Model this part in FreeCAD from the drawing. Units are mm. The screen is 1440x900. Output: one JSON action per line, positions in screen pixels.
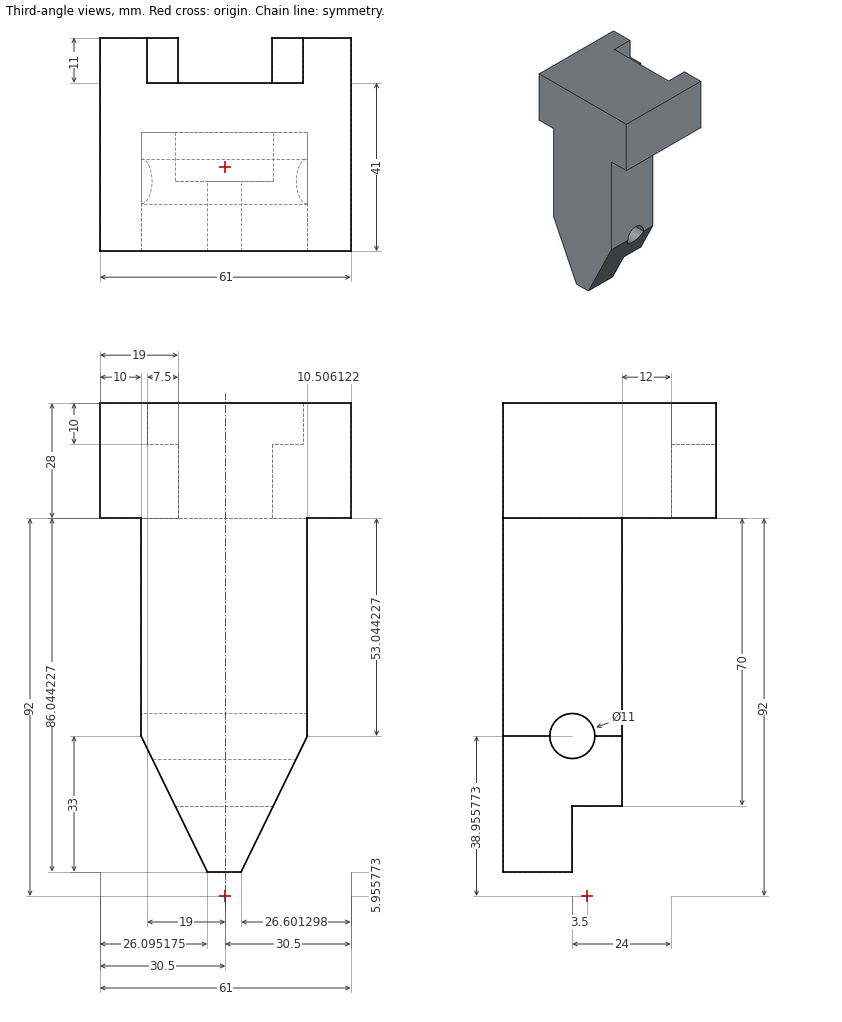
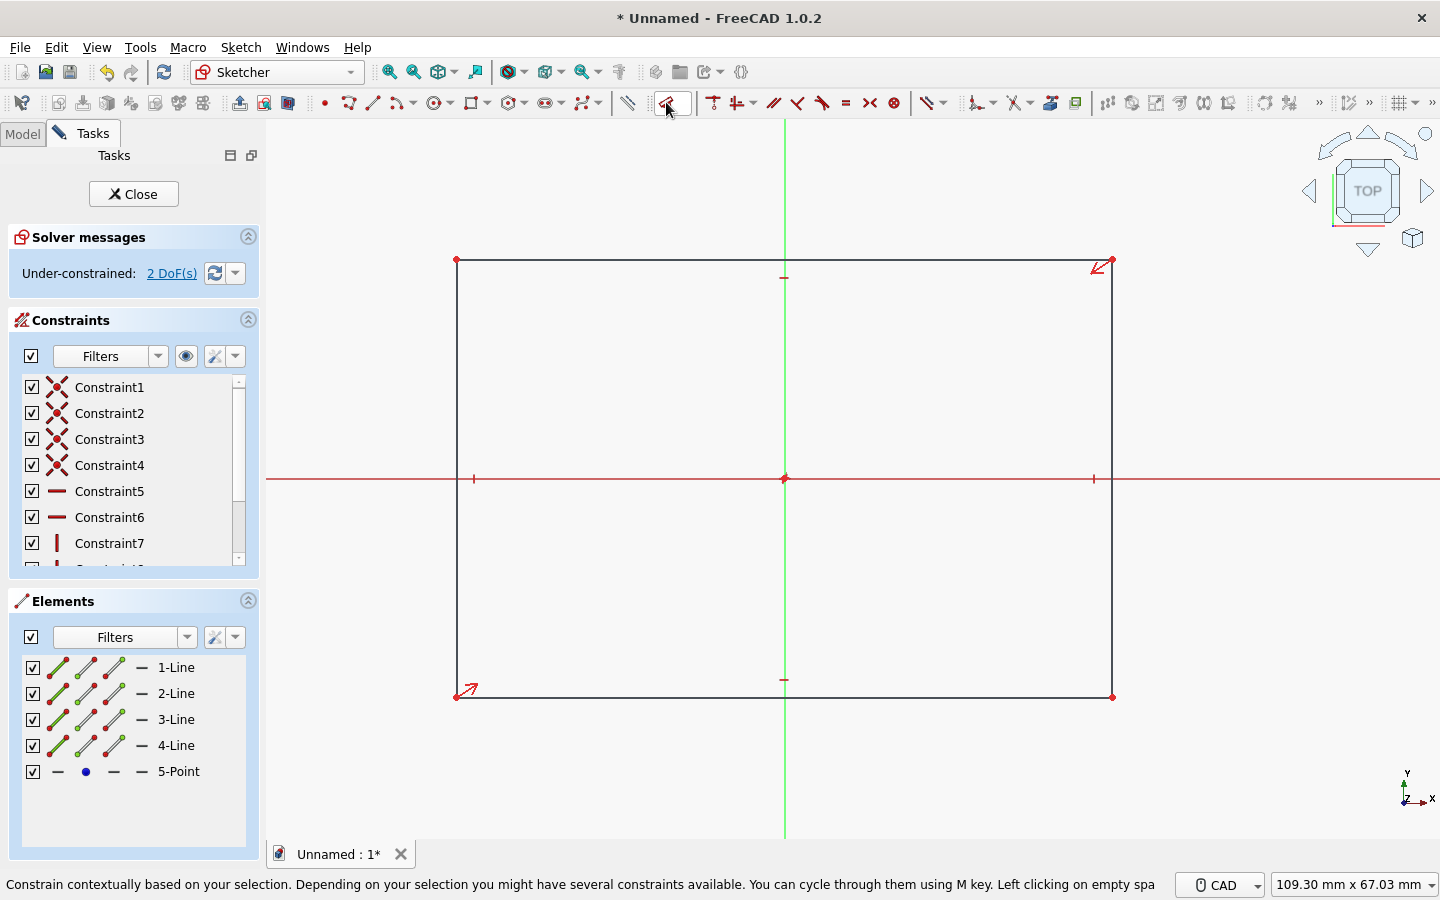
{"action": "left_click", "coordinate": [653, 698]}
{"action": "left_click", "coordinate": [634, 732]}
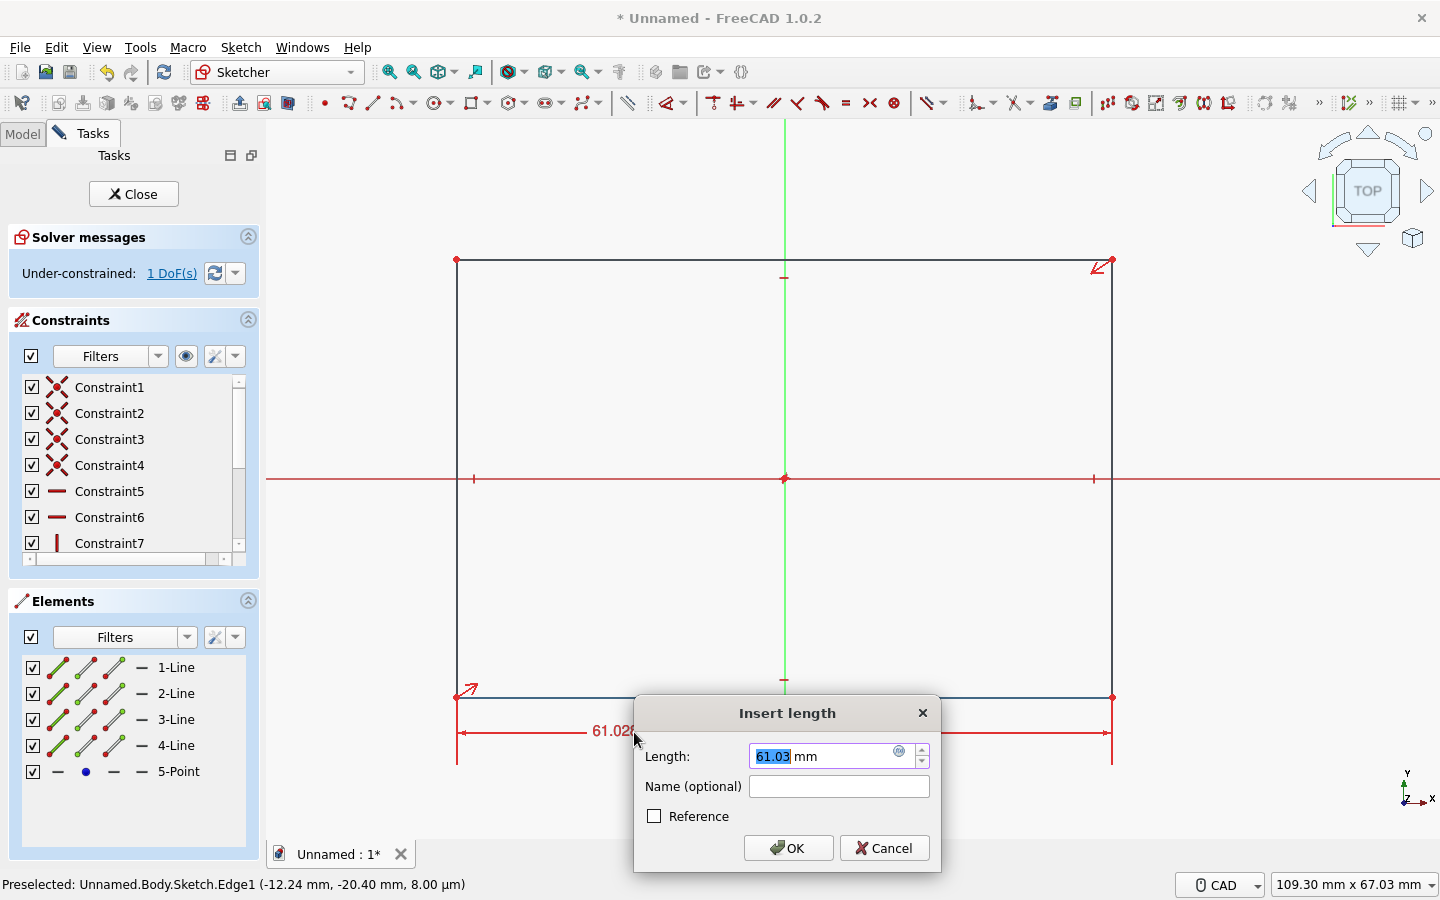
{"action": "type", "text": "61"}
{"action": "key", "text": "Return"}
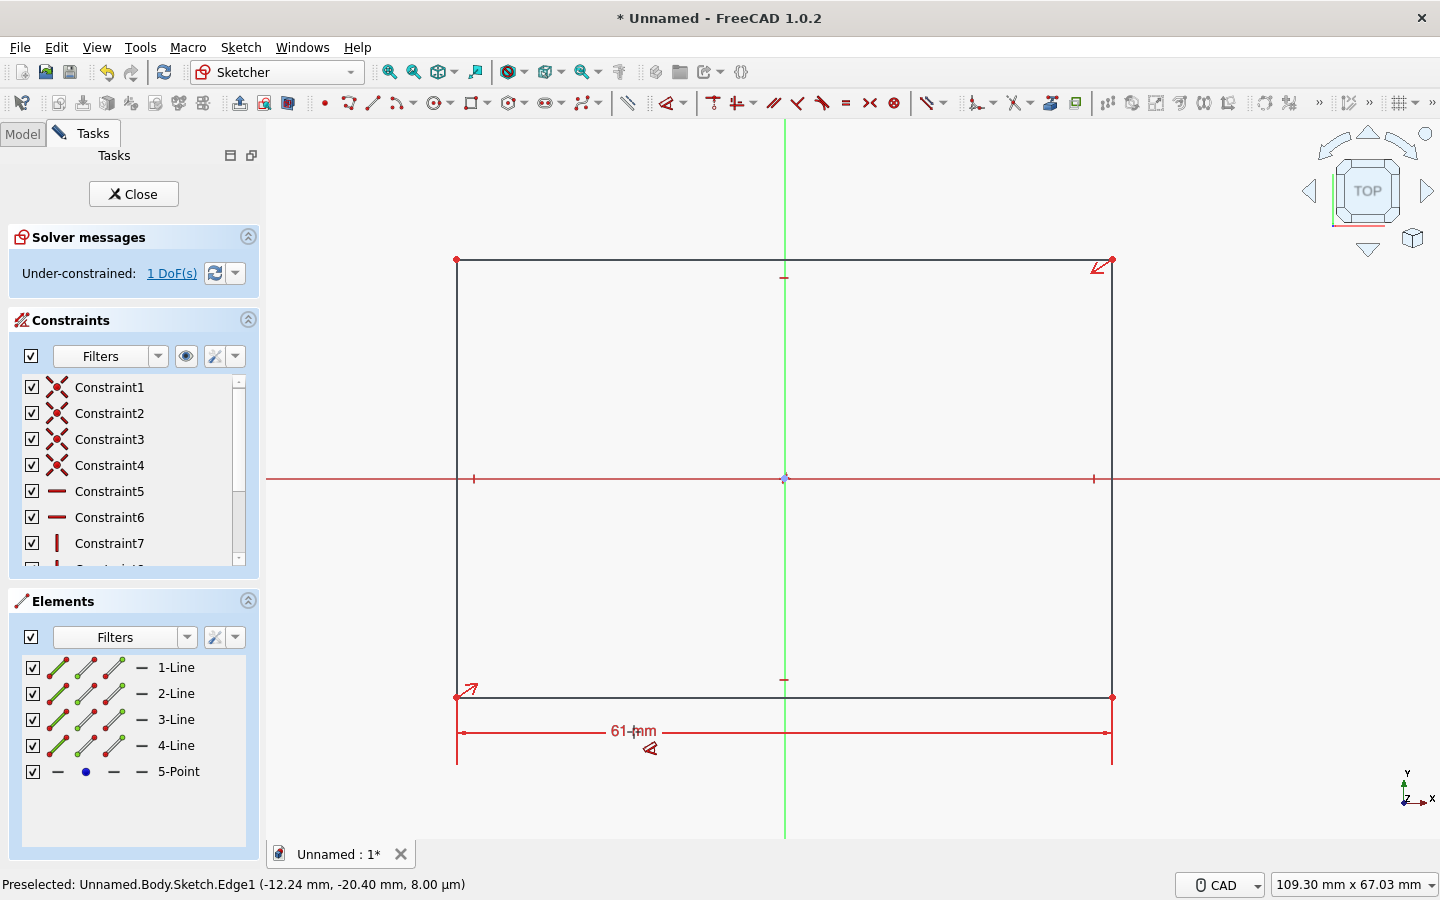
{"action": "left_click", "coordinate": [1112, 566]}
{"action": "left_click", "coordinate": [1146, 378]}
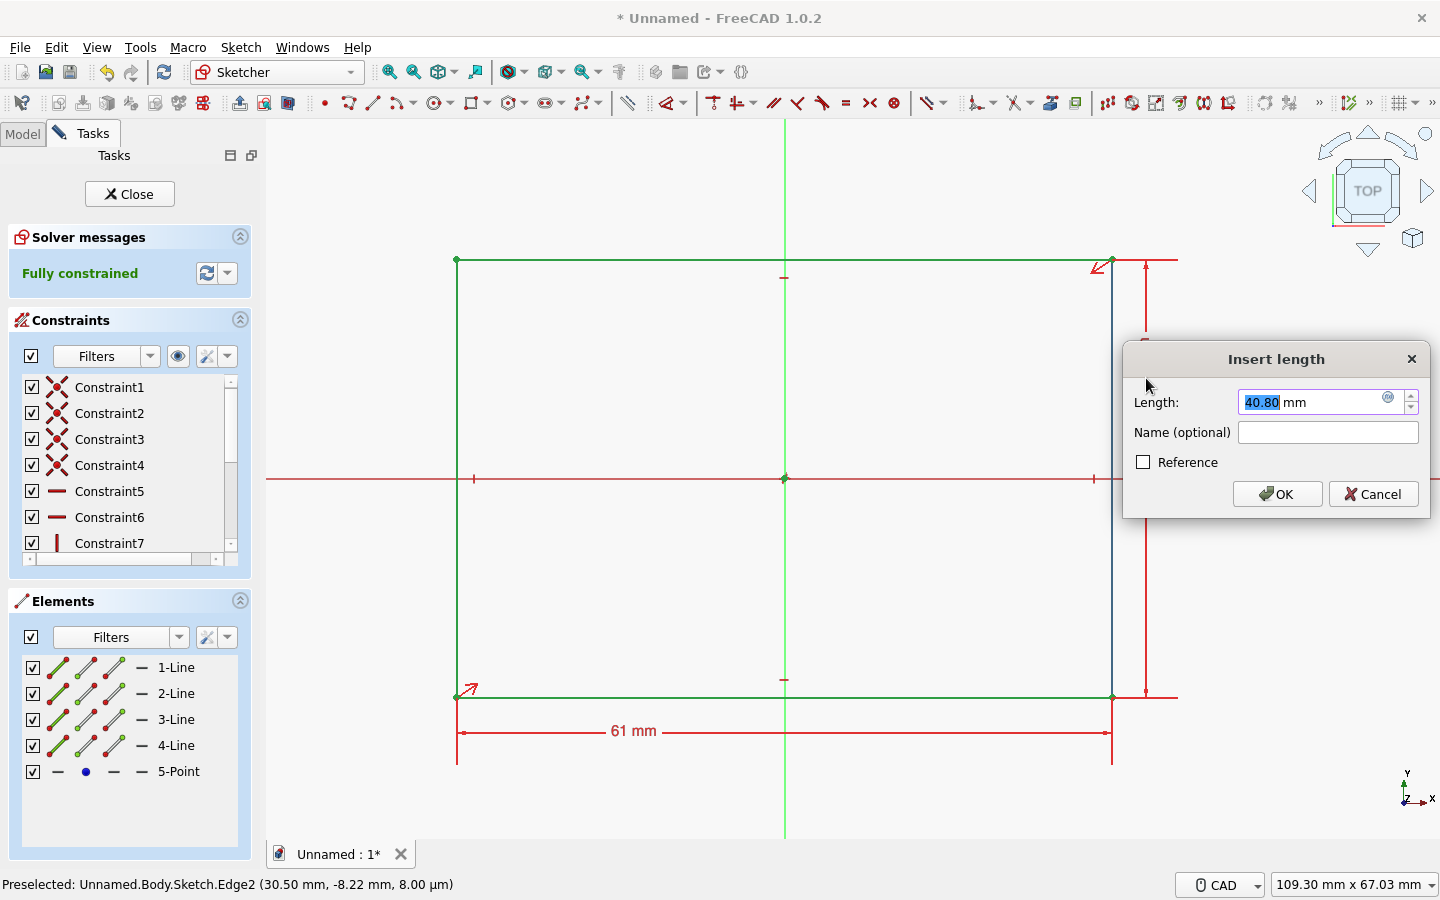
{"action": "type", "text": "41"}
{"action": "key", "text": "Return"}
{"action": "key", "text": "Escape"}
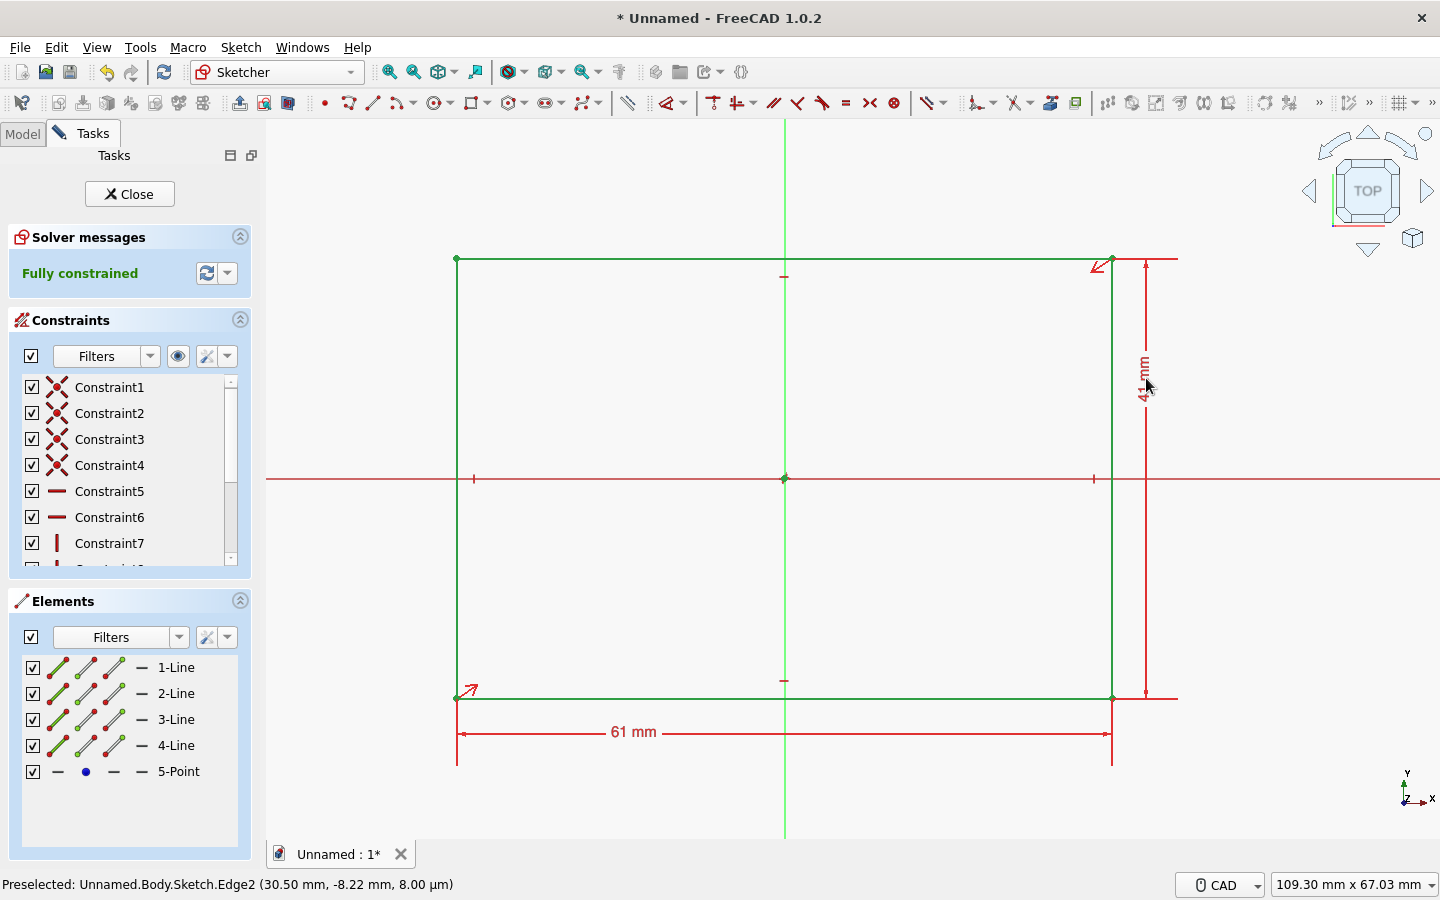
{"action": "left_click", "coordinate": [130, 194]}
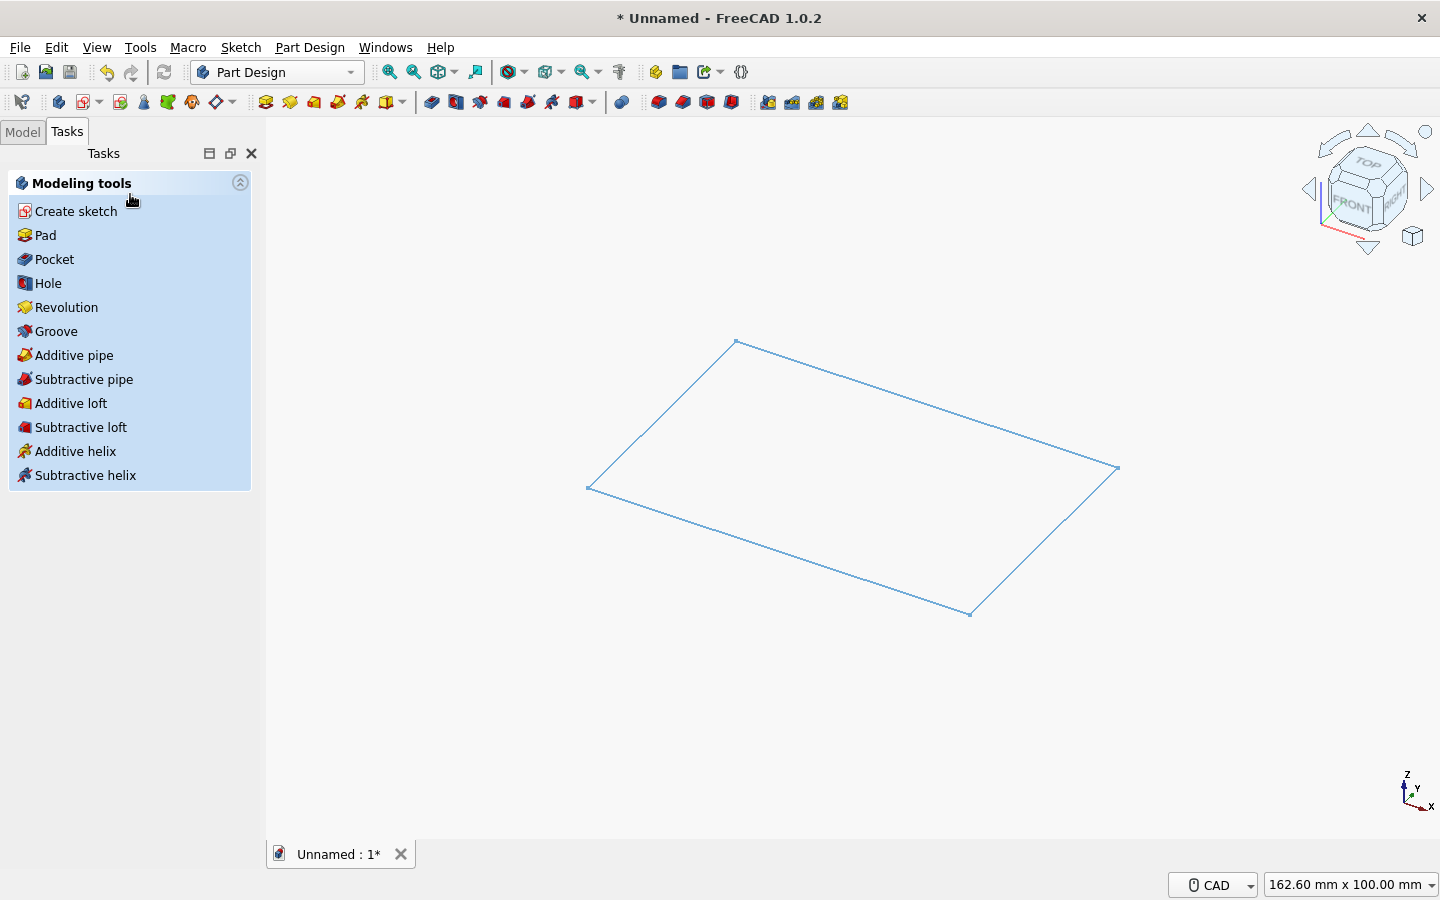
{"action": "left_click", "coordinate": [266, 102]}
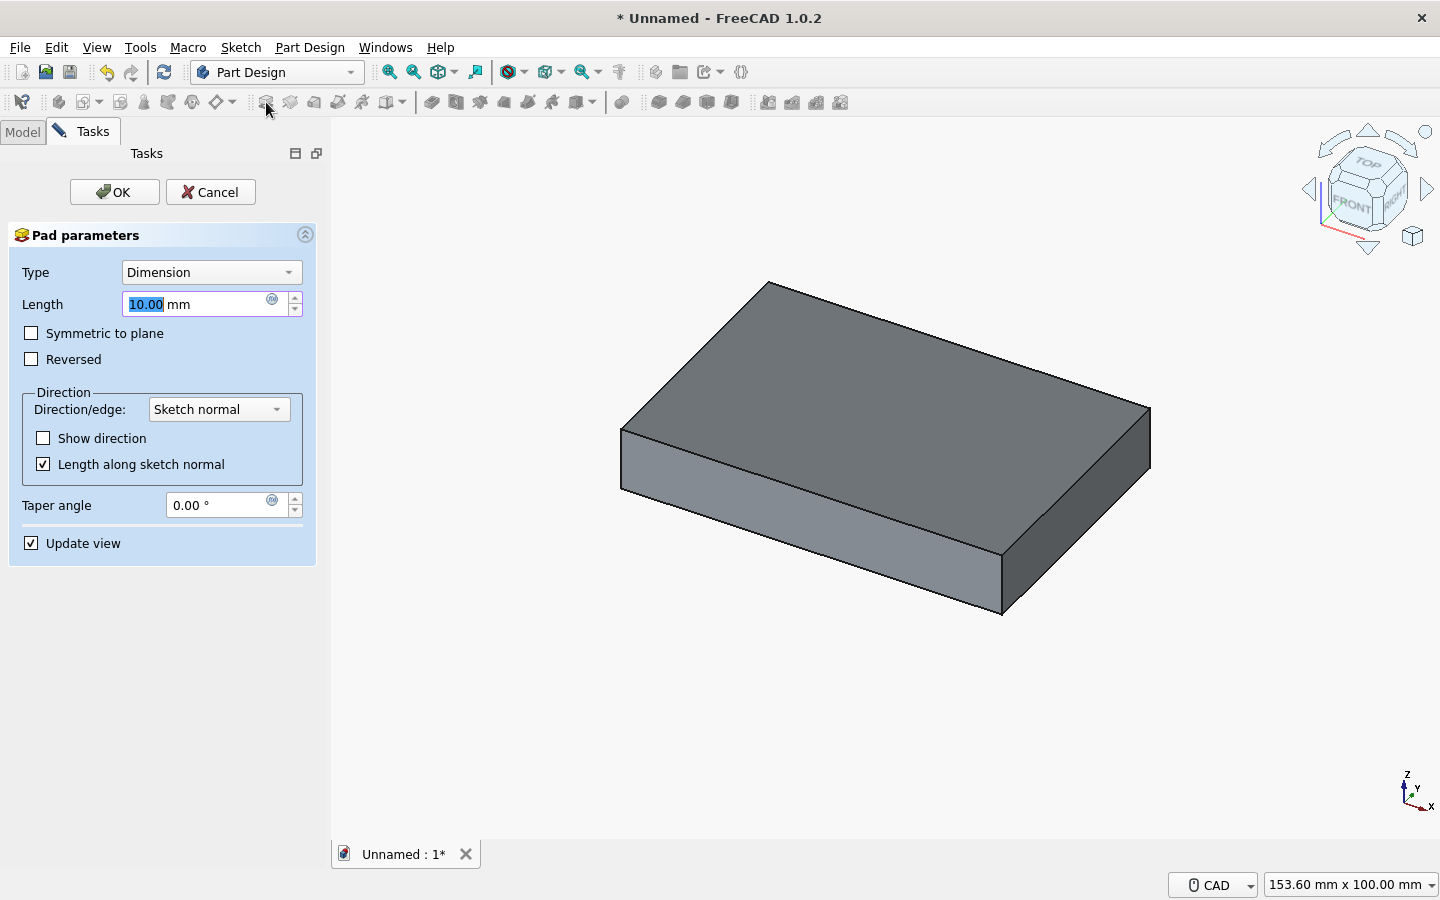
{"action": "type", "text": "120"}
{"action": "key", "text": "Tab"}